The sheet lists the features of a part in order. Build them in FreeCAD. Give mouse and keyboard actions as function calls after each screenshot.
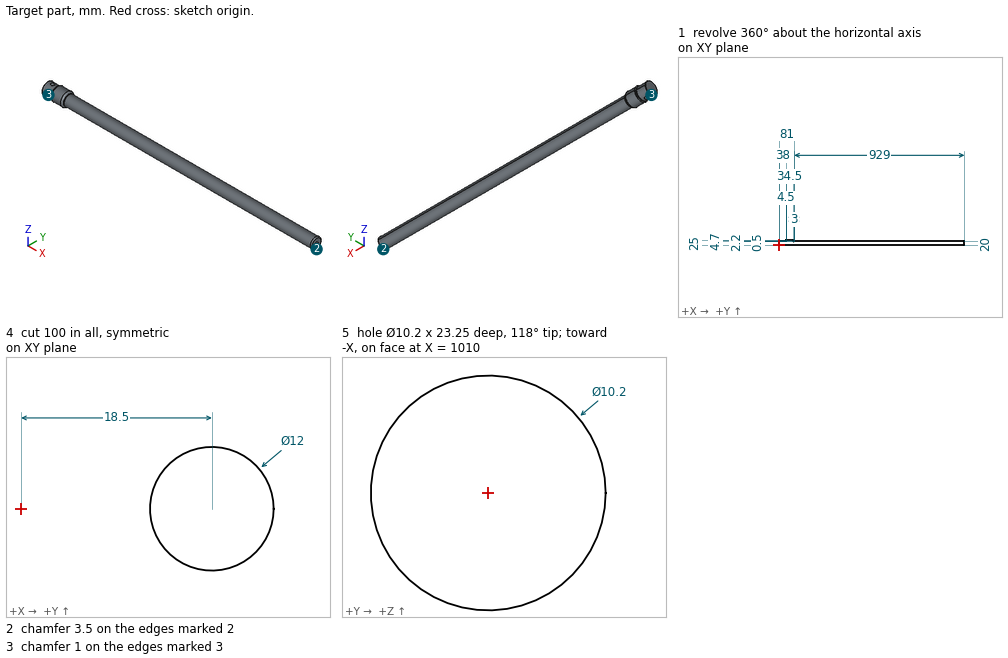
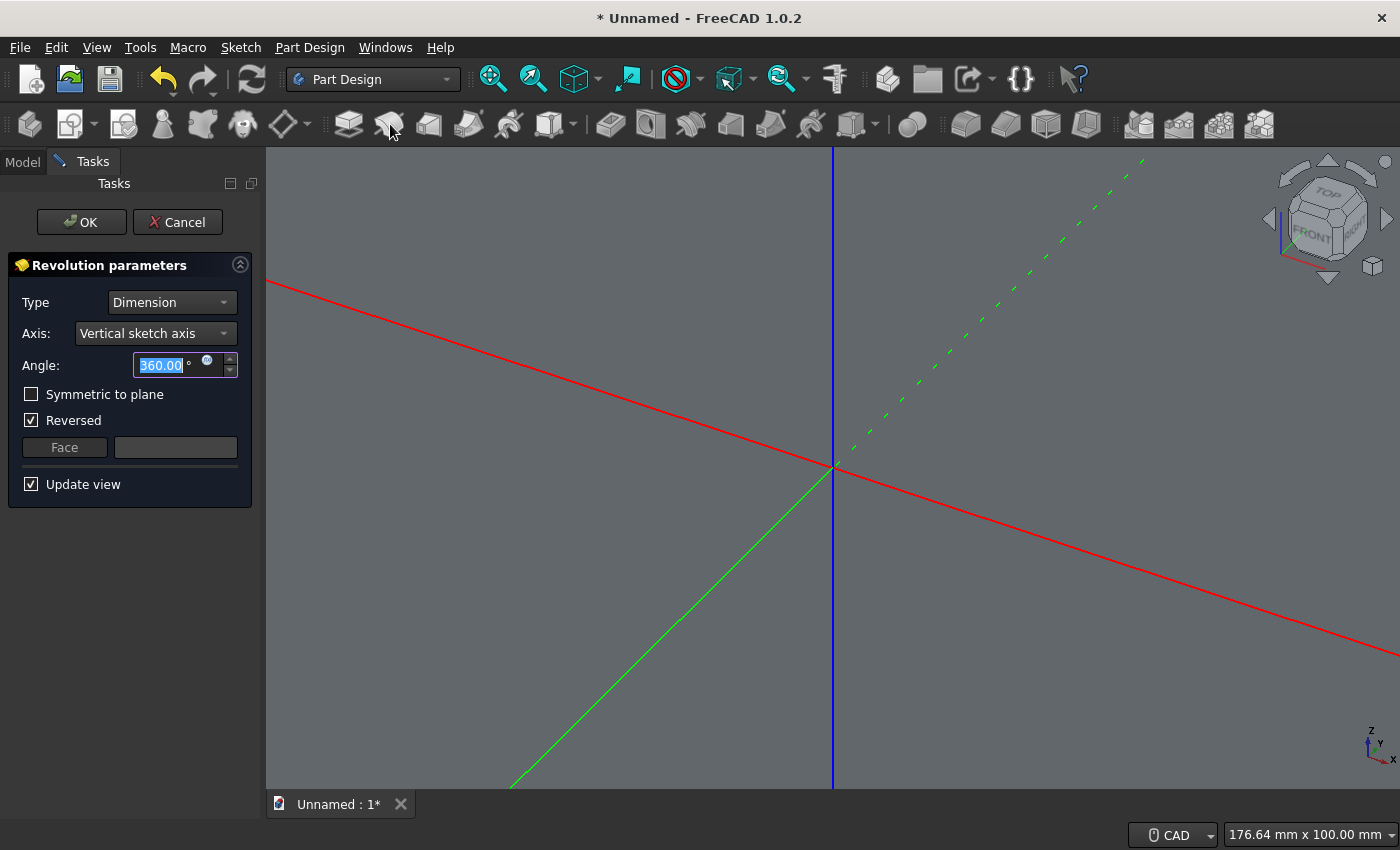
click(156, 334)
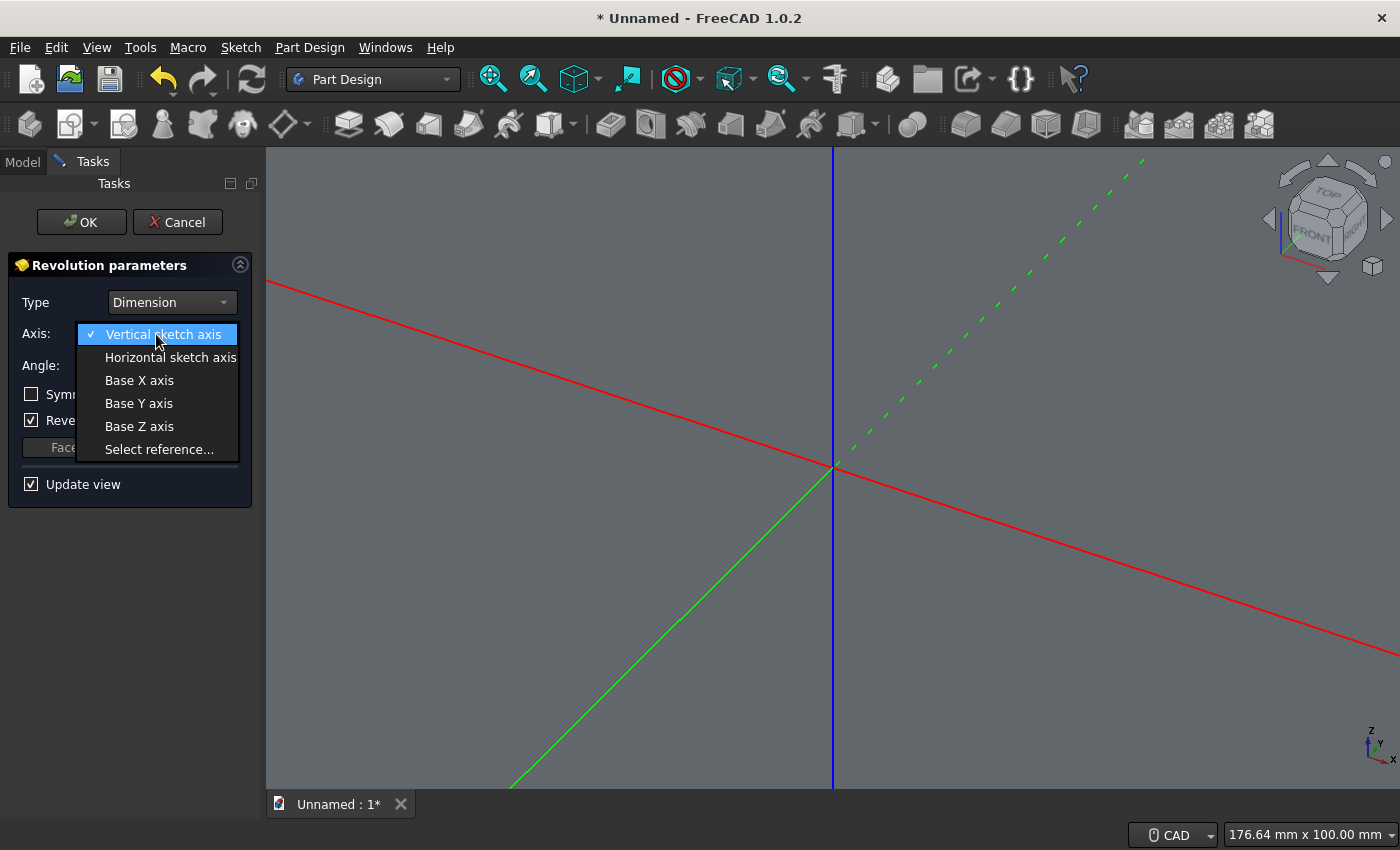
click(156, 358)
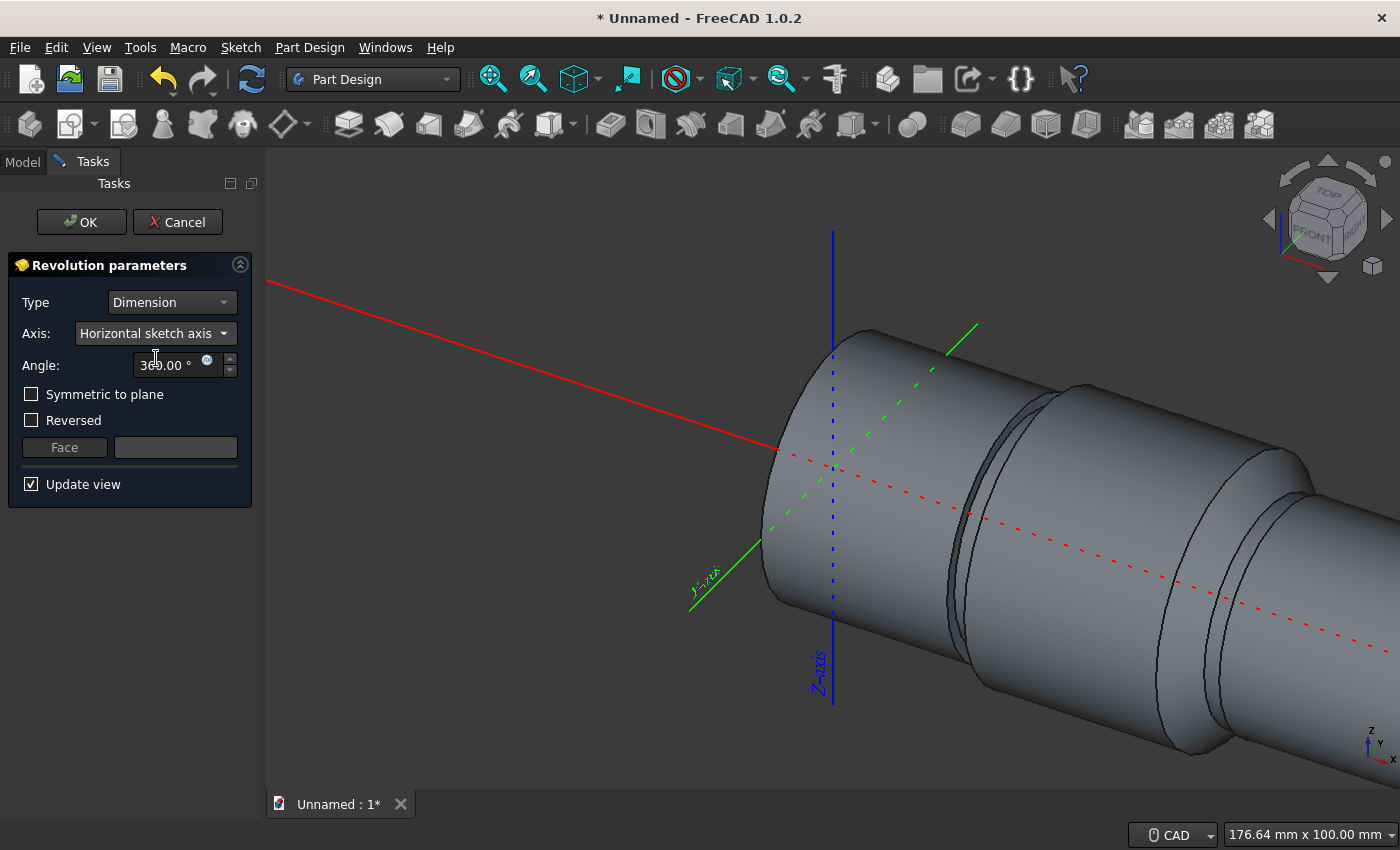
click(82, 222)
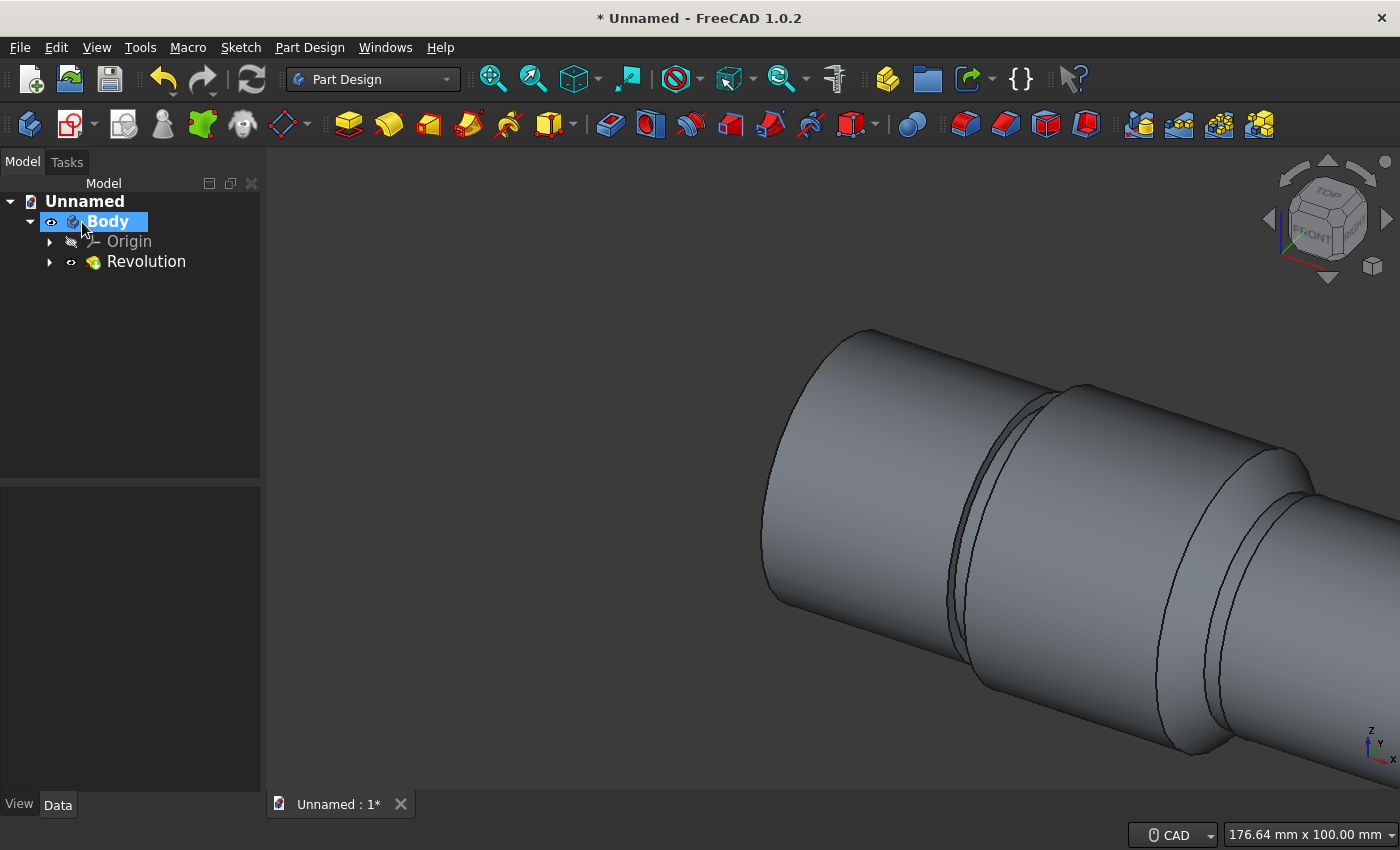
click(494, 80)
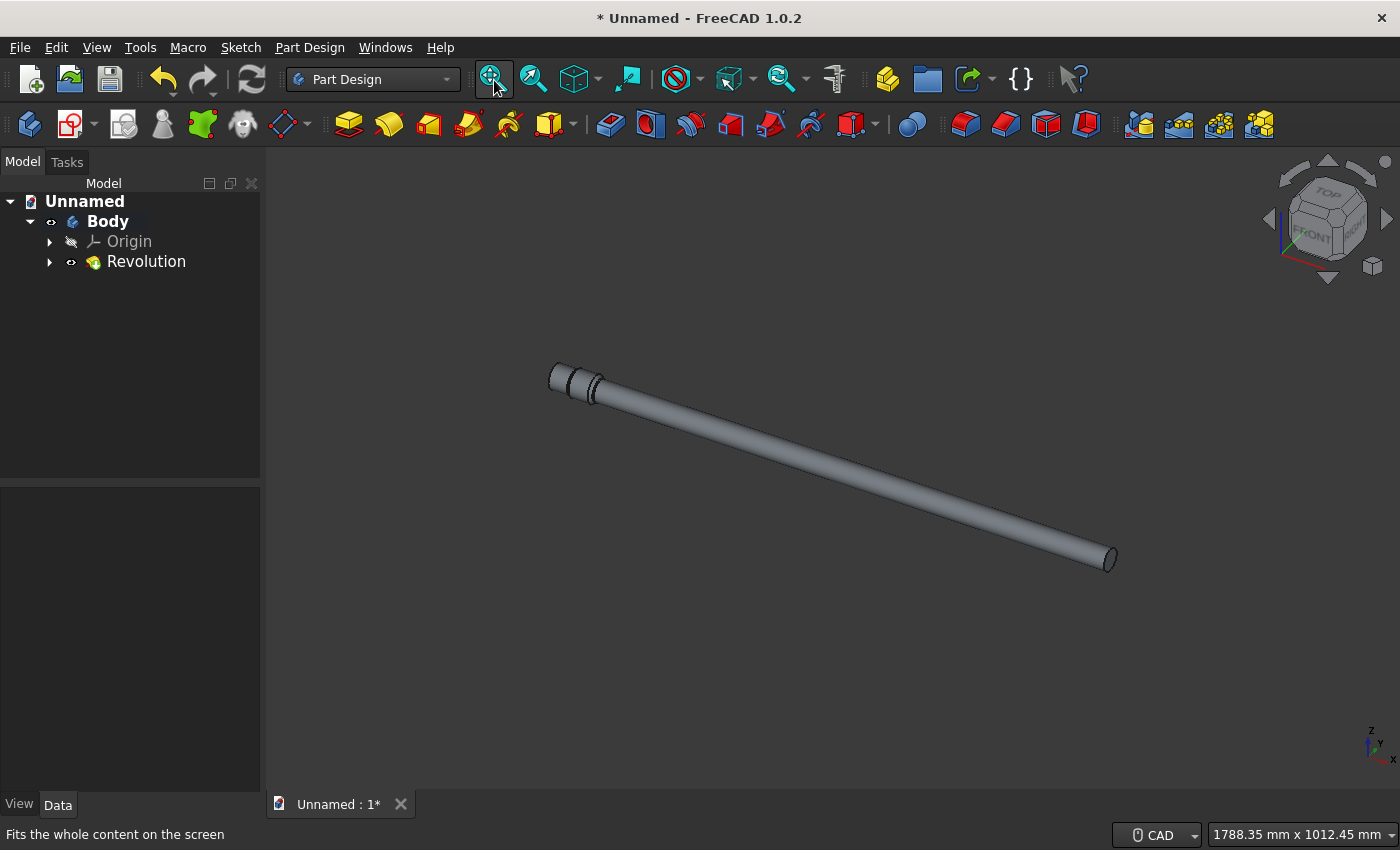
click(1104, 565)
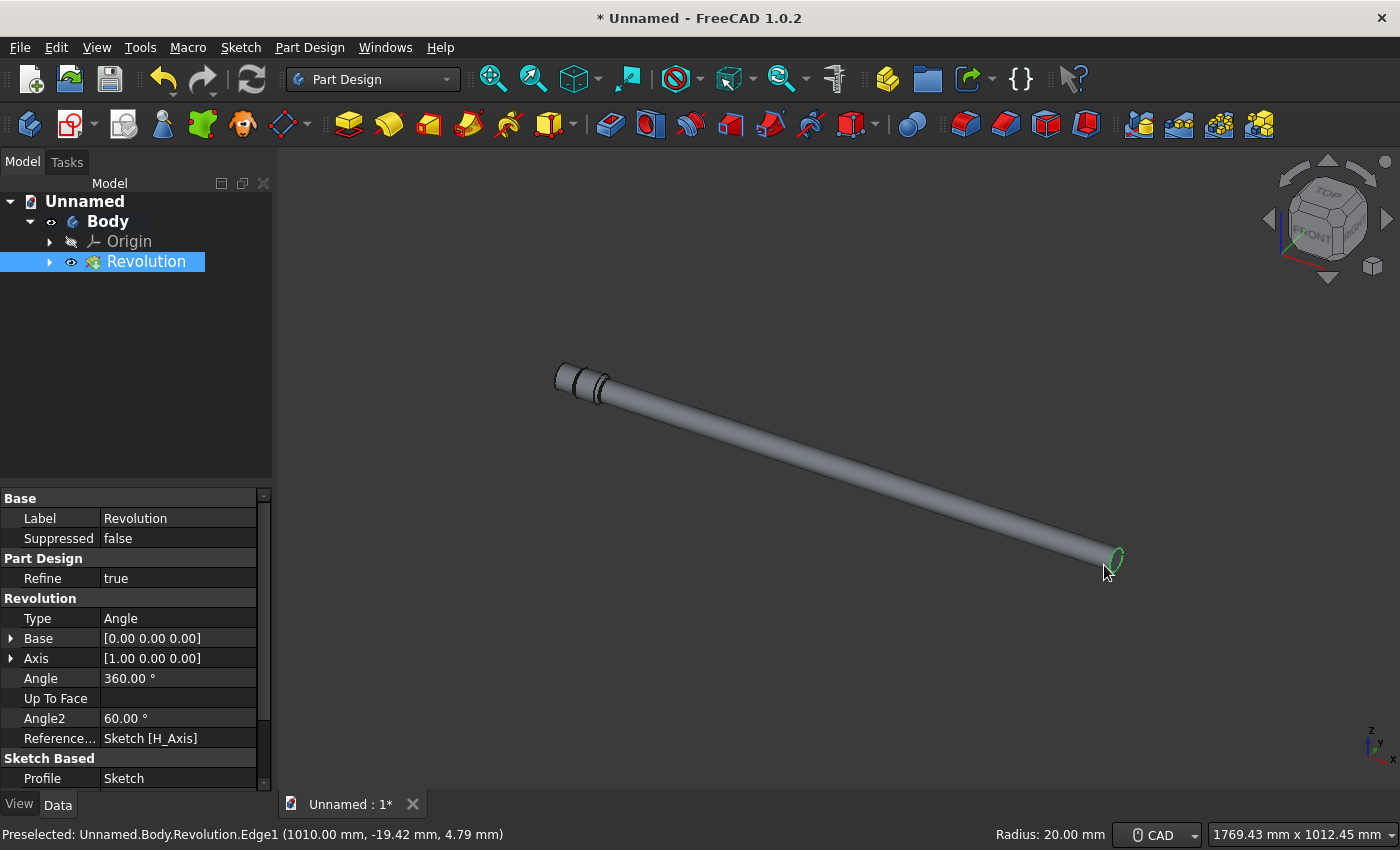
click(1006, 124)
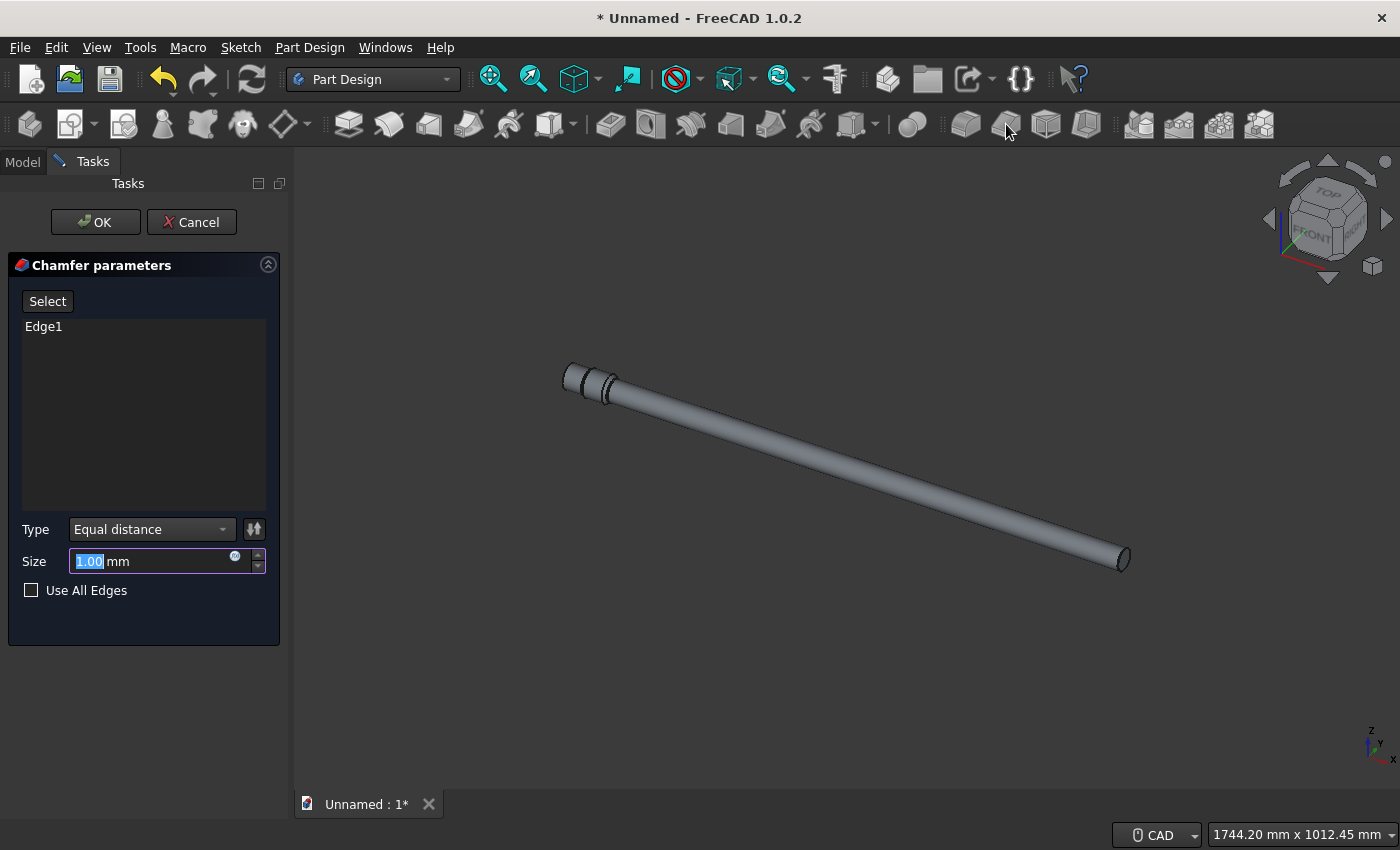
text(3.5)
key(Tab)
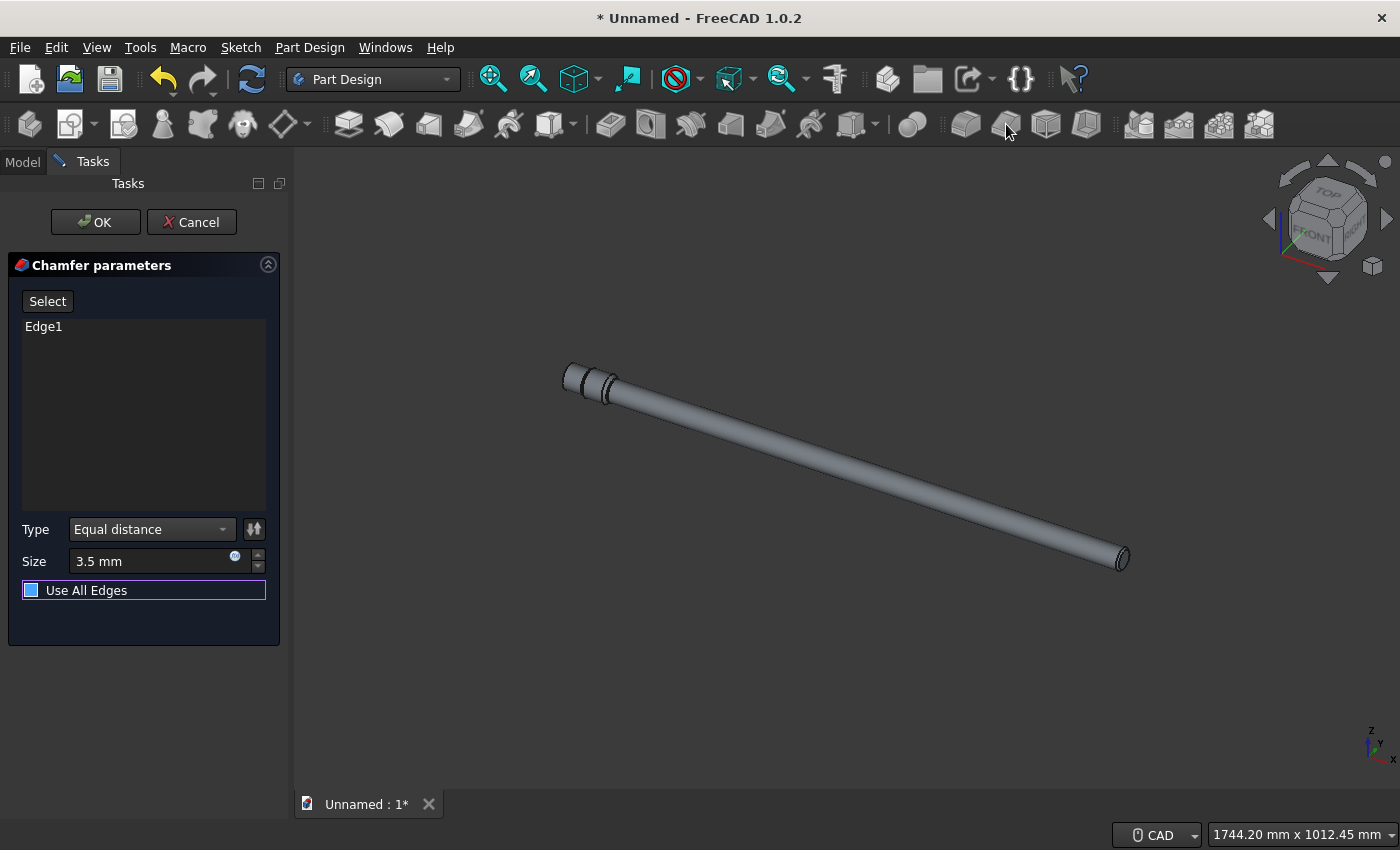
click(96, 222)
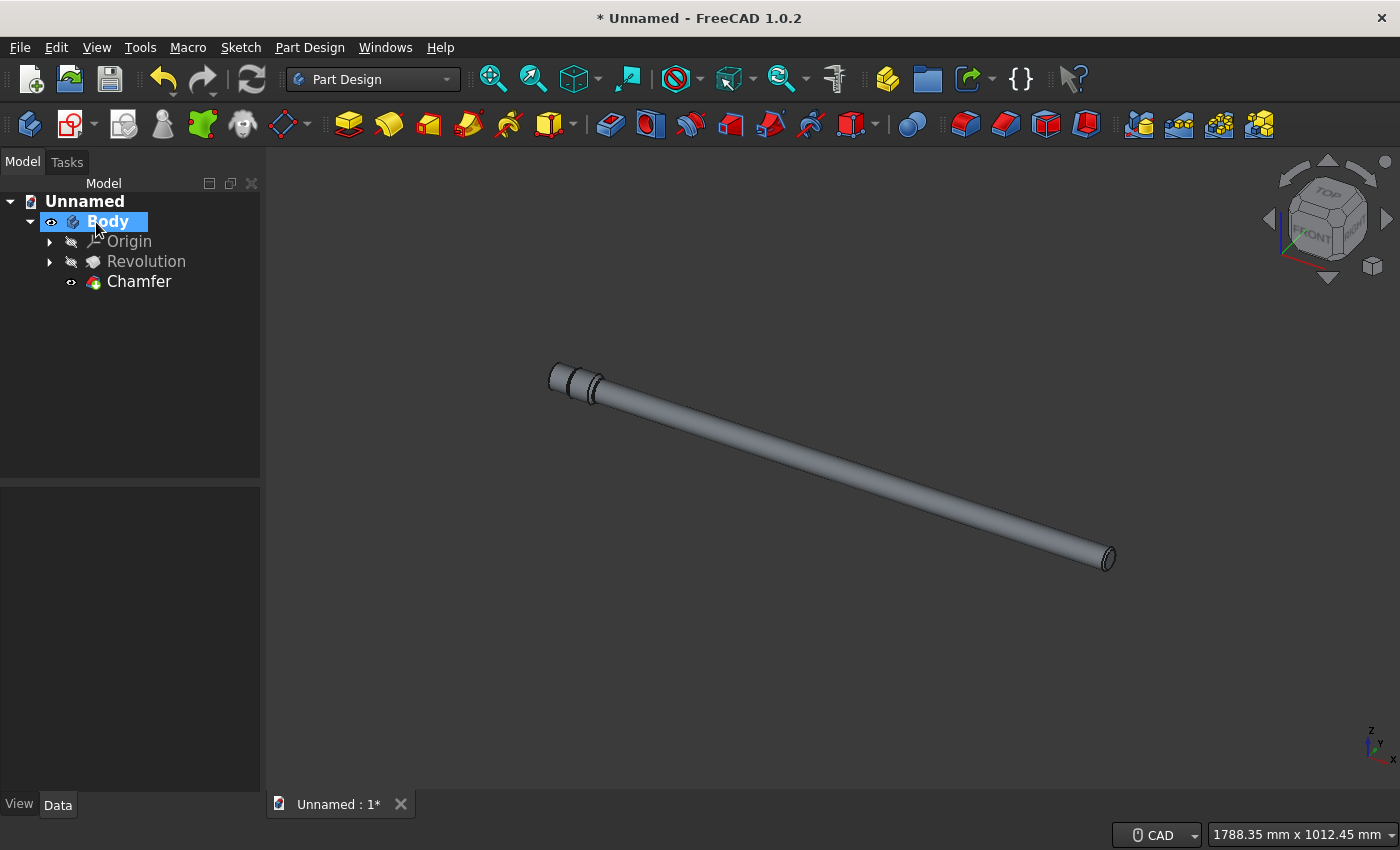
click(549, 382)